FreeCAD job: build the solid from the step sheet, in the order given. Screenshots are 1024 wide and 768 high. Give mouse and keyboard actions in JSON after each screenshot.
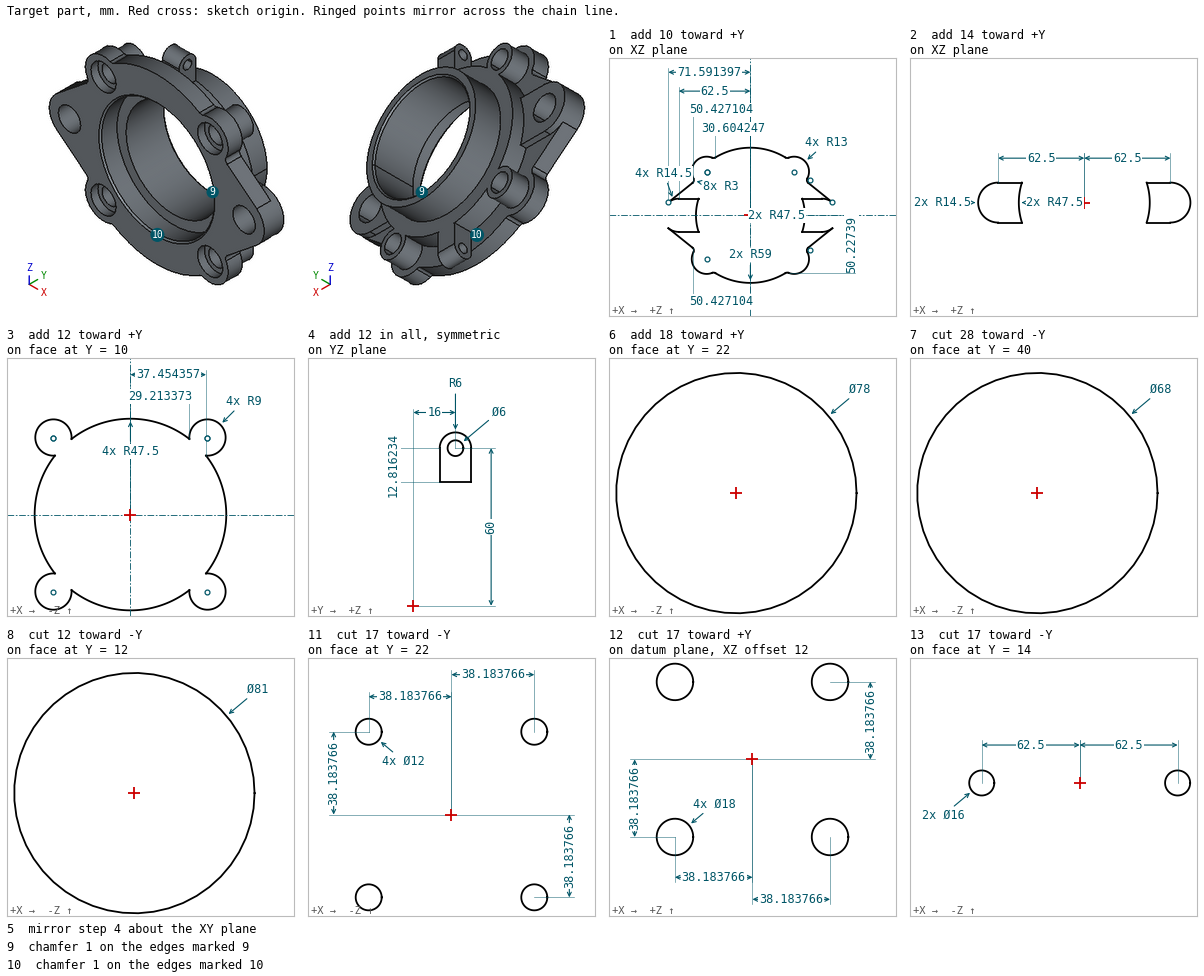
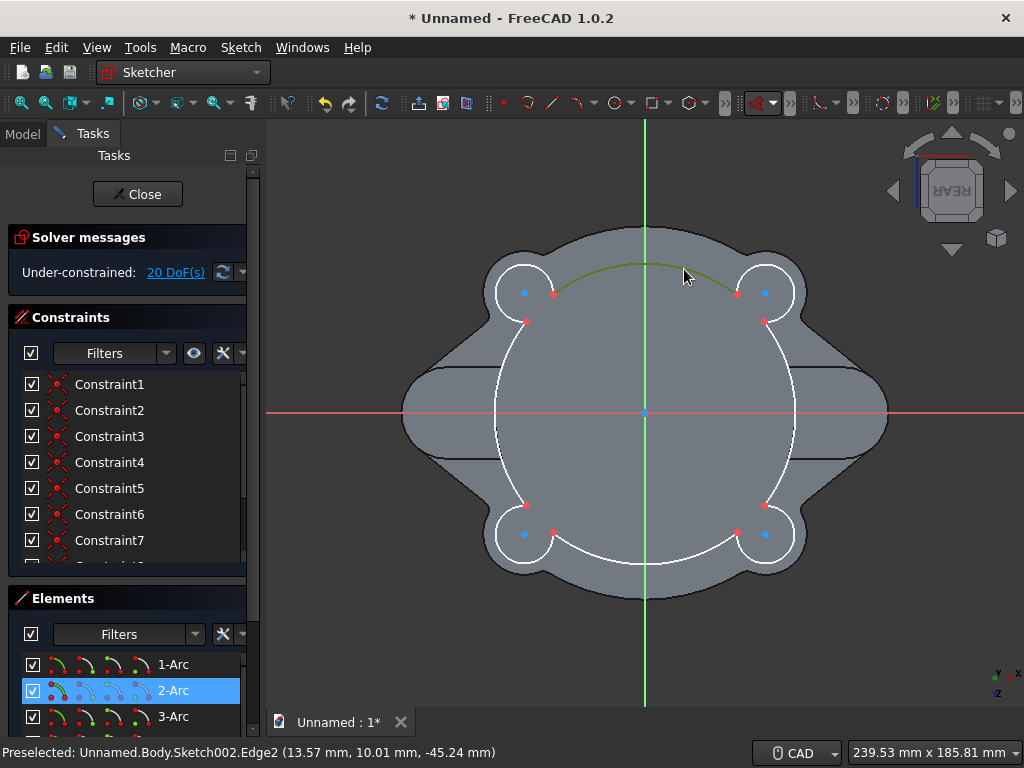
{"action": "left_click", "coordinate": [790, 453]}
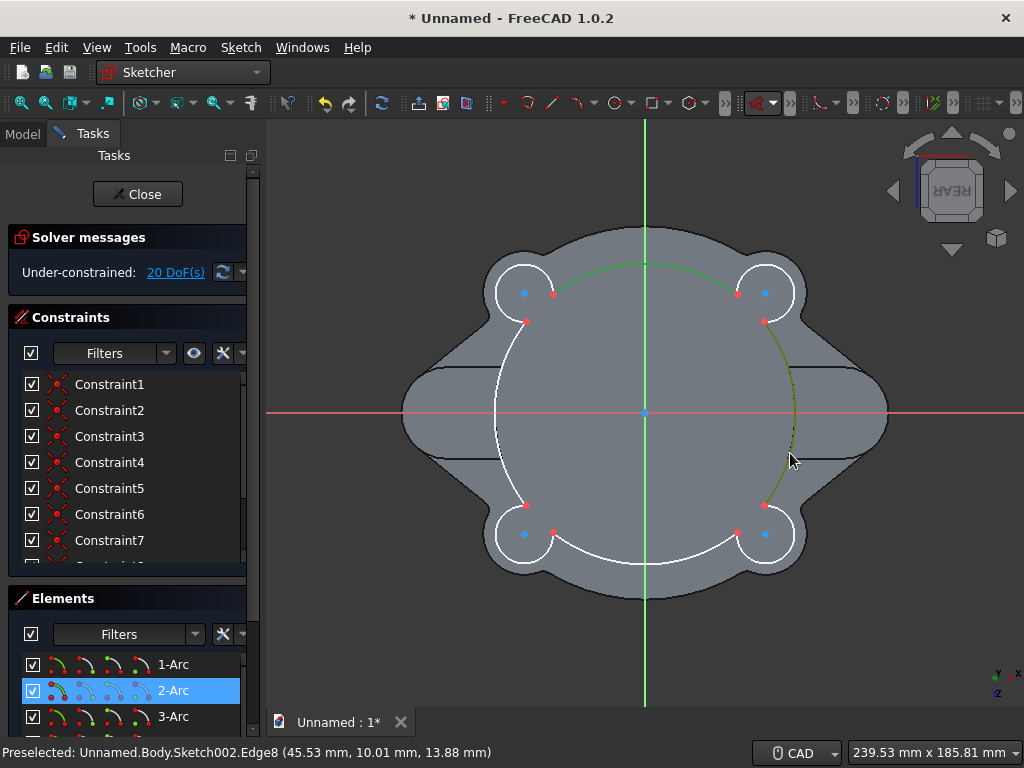
{"action": "key", "text": "c"}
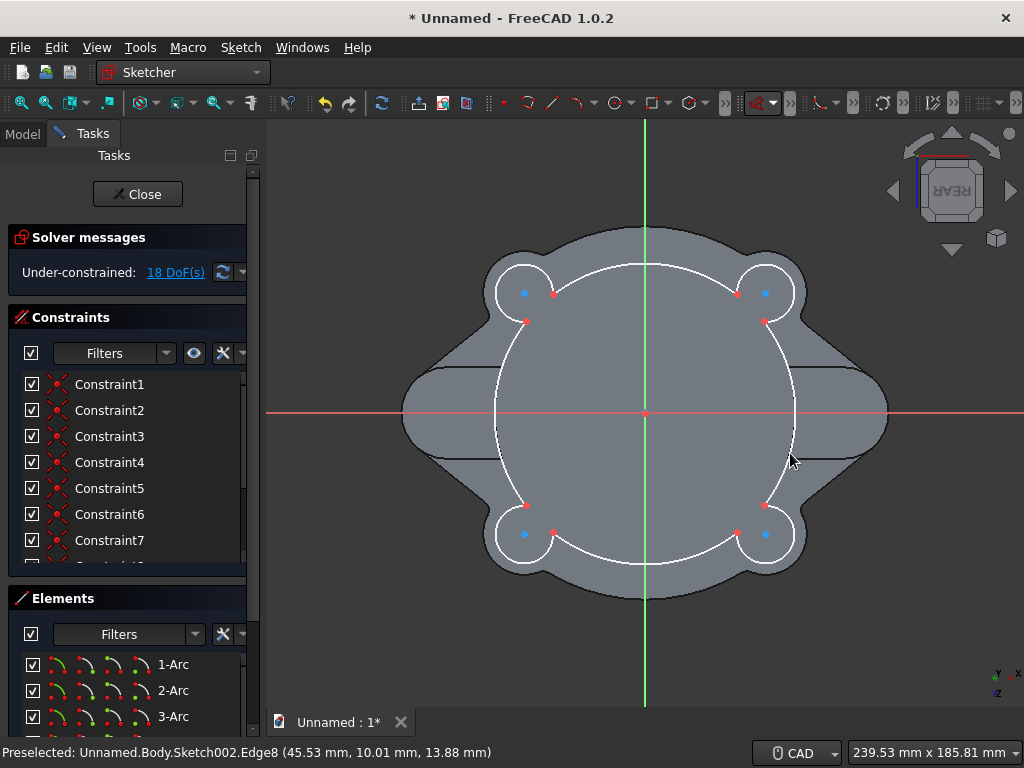
{"action": "scroll", "coordinate": [645, 413], "scroll_direction": "up", "scroll_amount": 2}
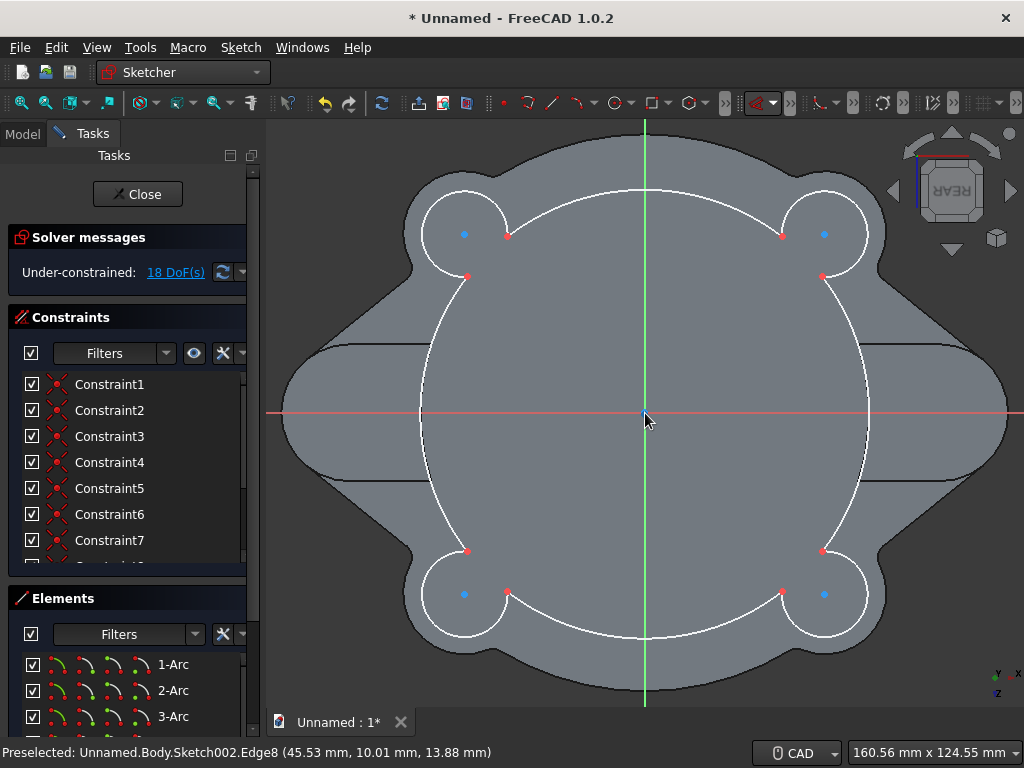
{"action": "left_click_drag", "start_coordinate": [635, 403], "coordinate": [655, 424]}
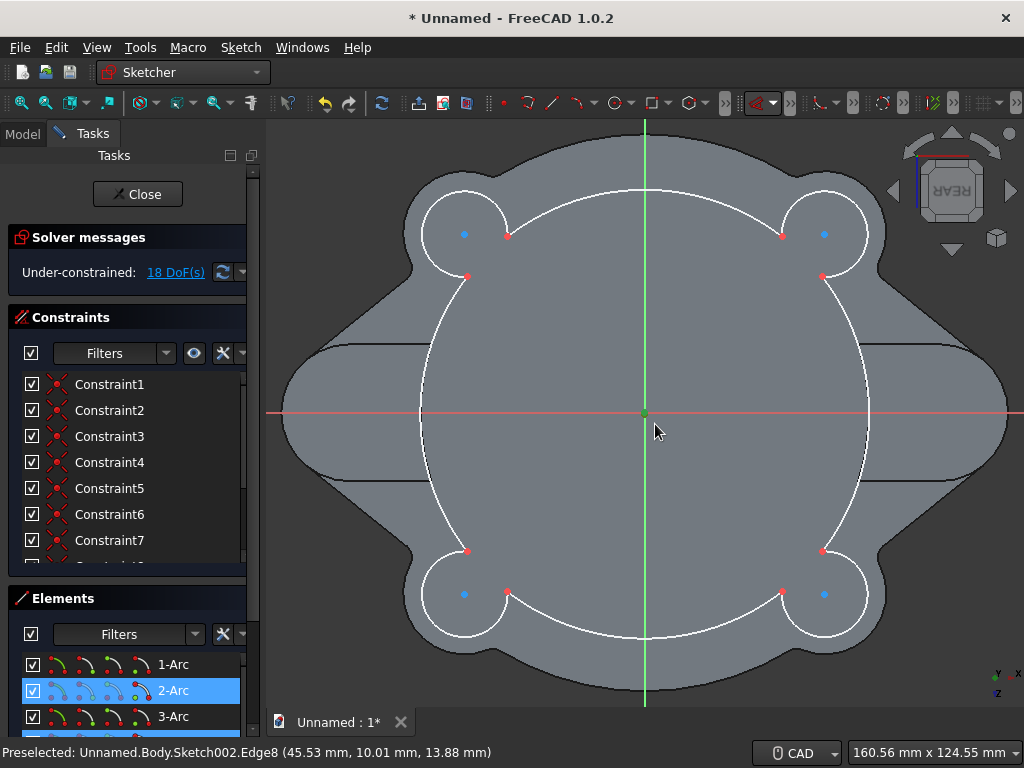
{"action": "key", "text": "c"}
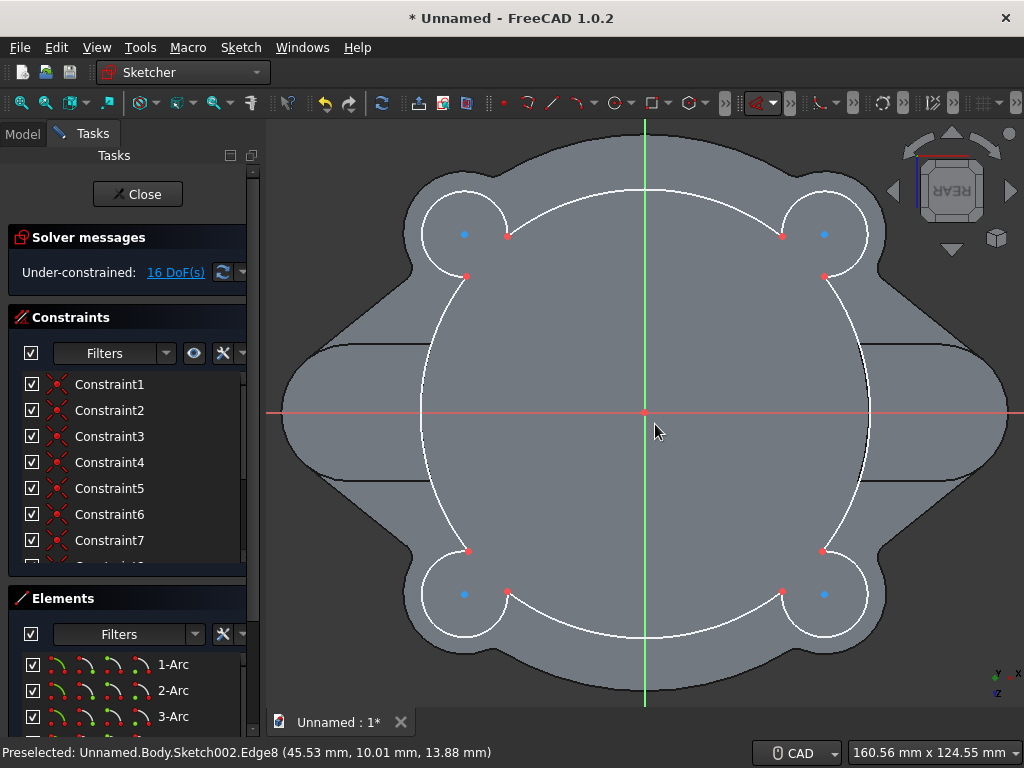
{"action": "left_click", "coordinate": [816, 192]}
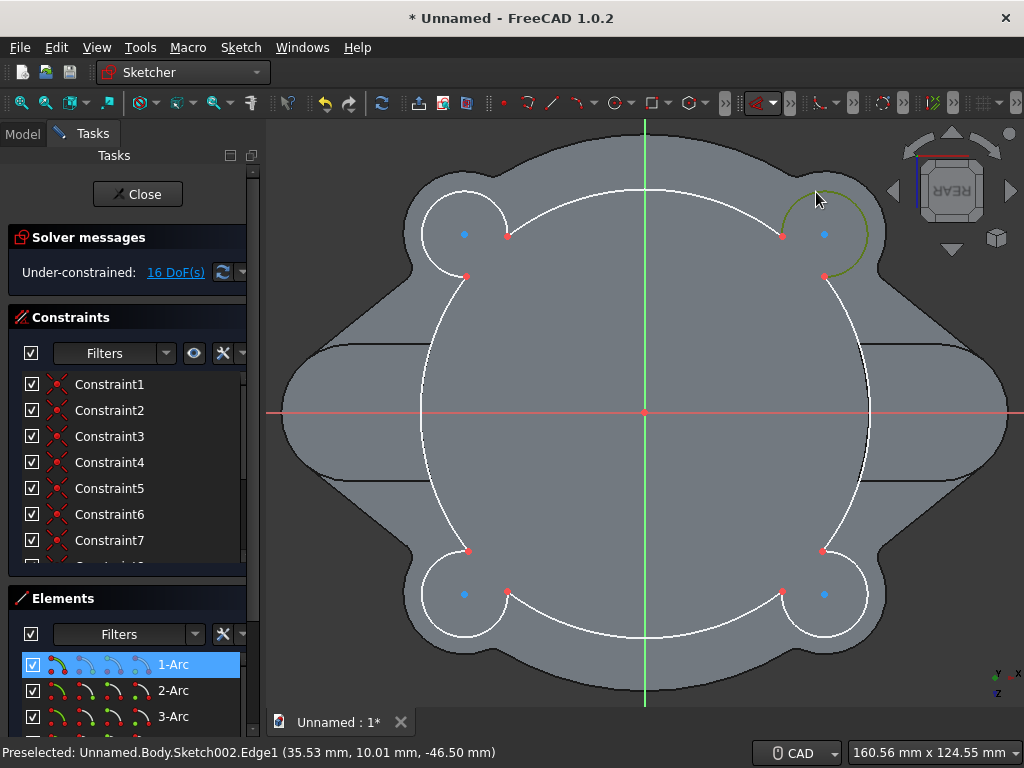
{"action": "left_click", "coordinate": [473, 192]}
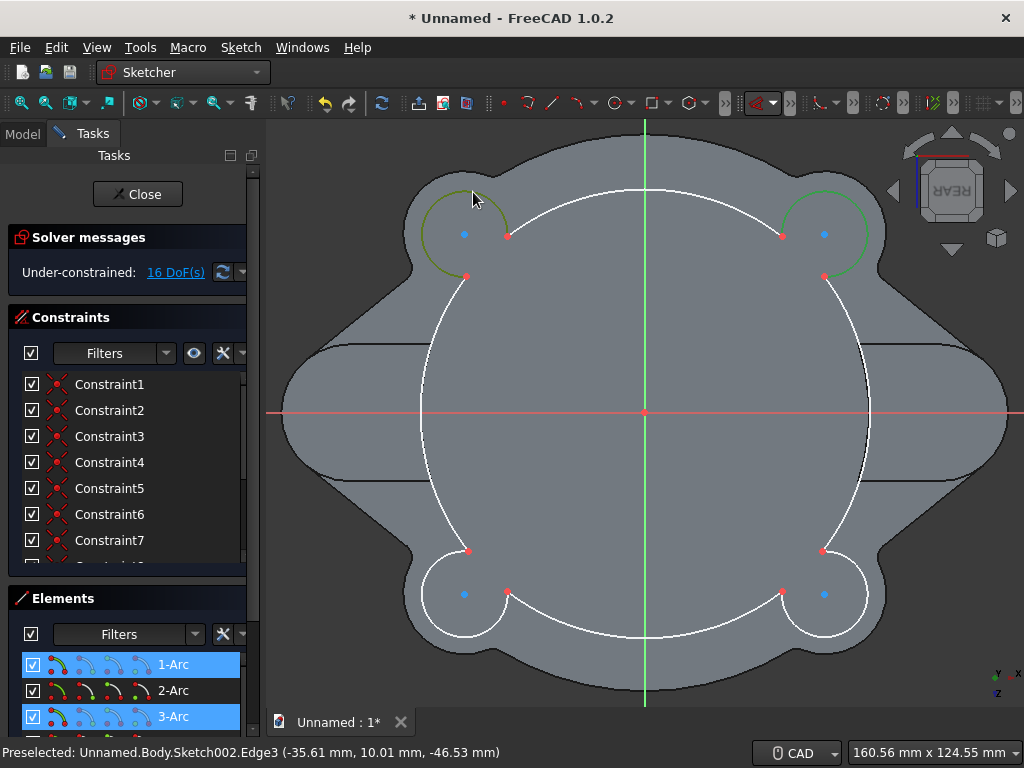
{"action": "left_click", "coordinate": [423, 586]}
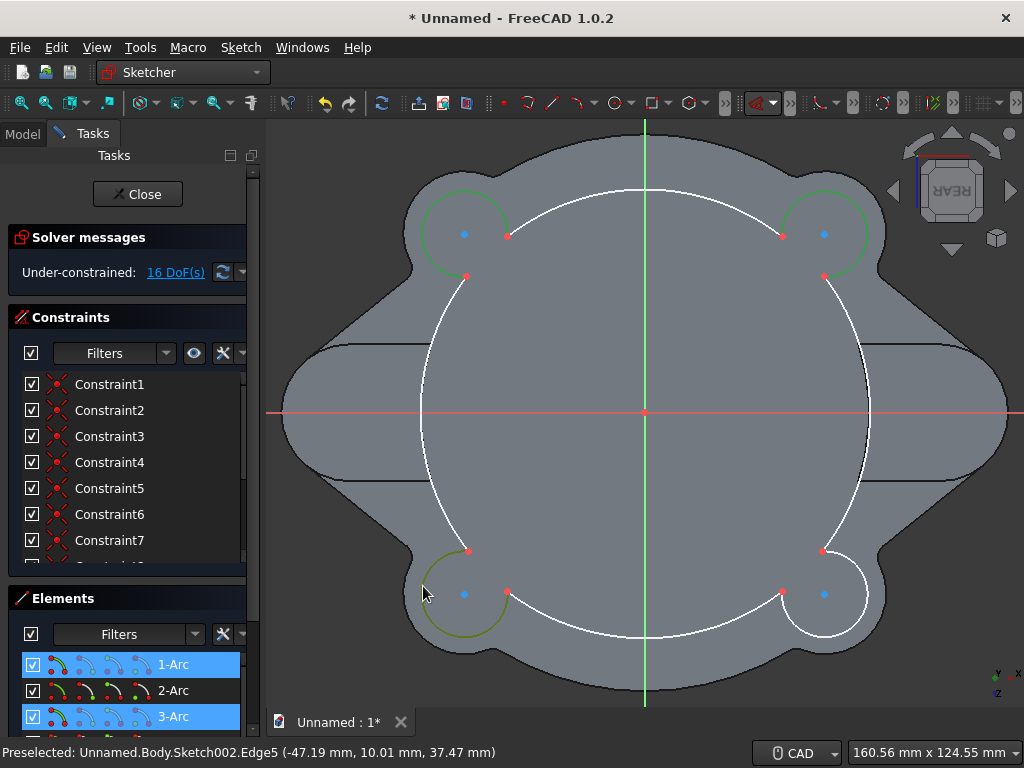
{"action": "left_click", "coordinate": [817, 636]}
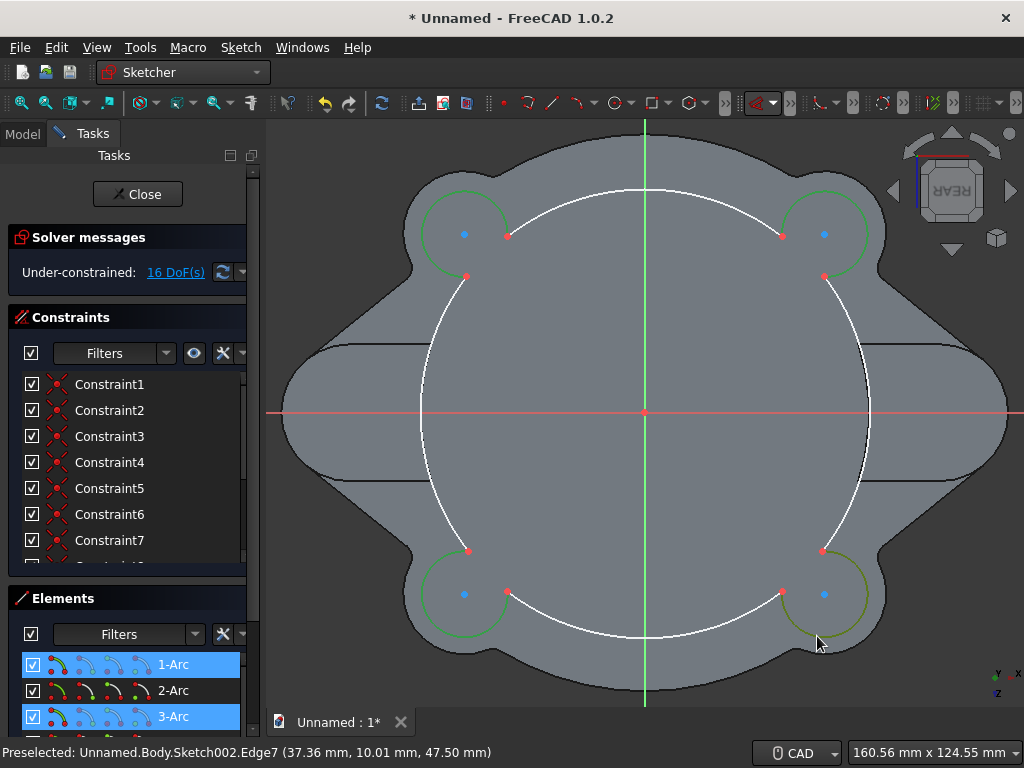
{"action": "key", "text": "e"}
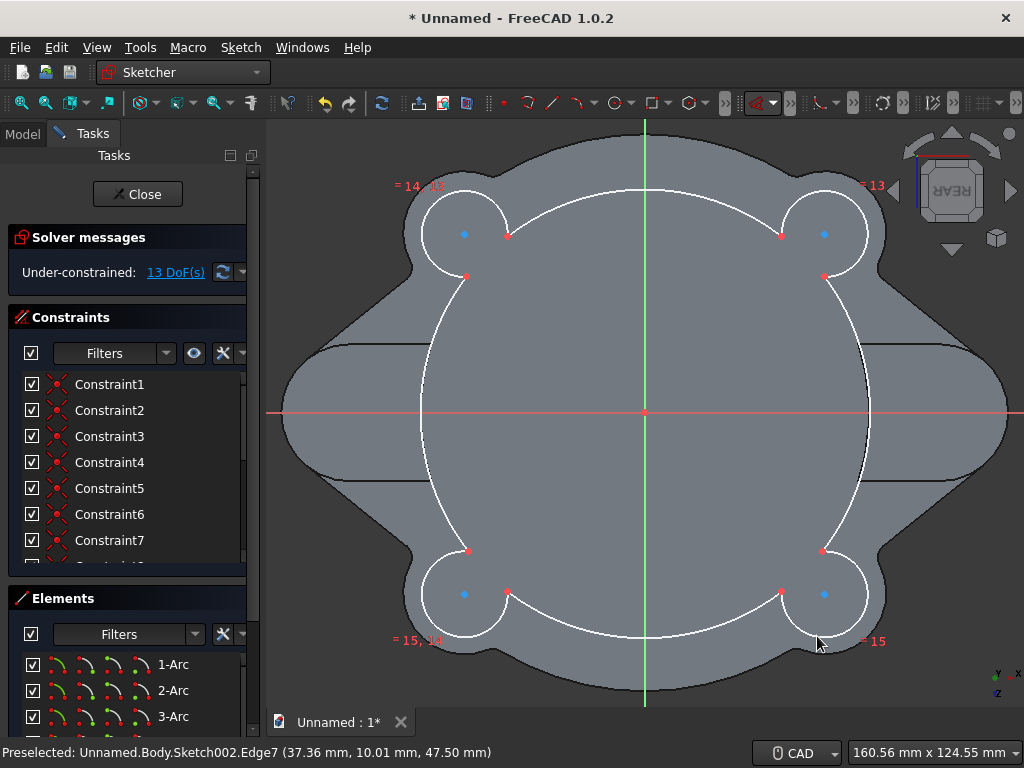
{"action": "left_click", "coordinate": [703, 197]}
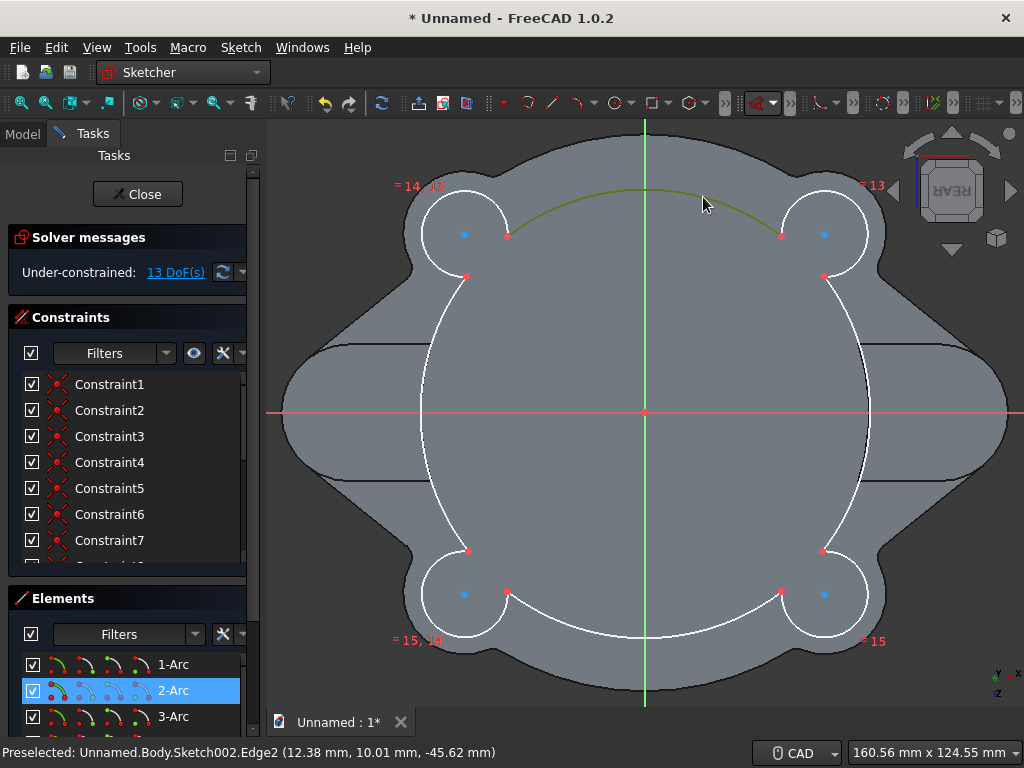
{"action": "left_click", "coordinate": [428, 356]}